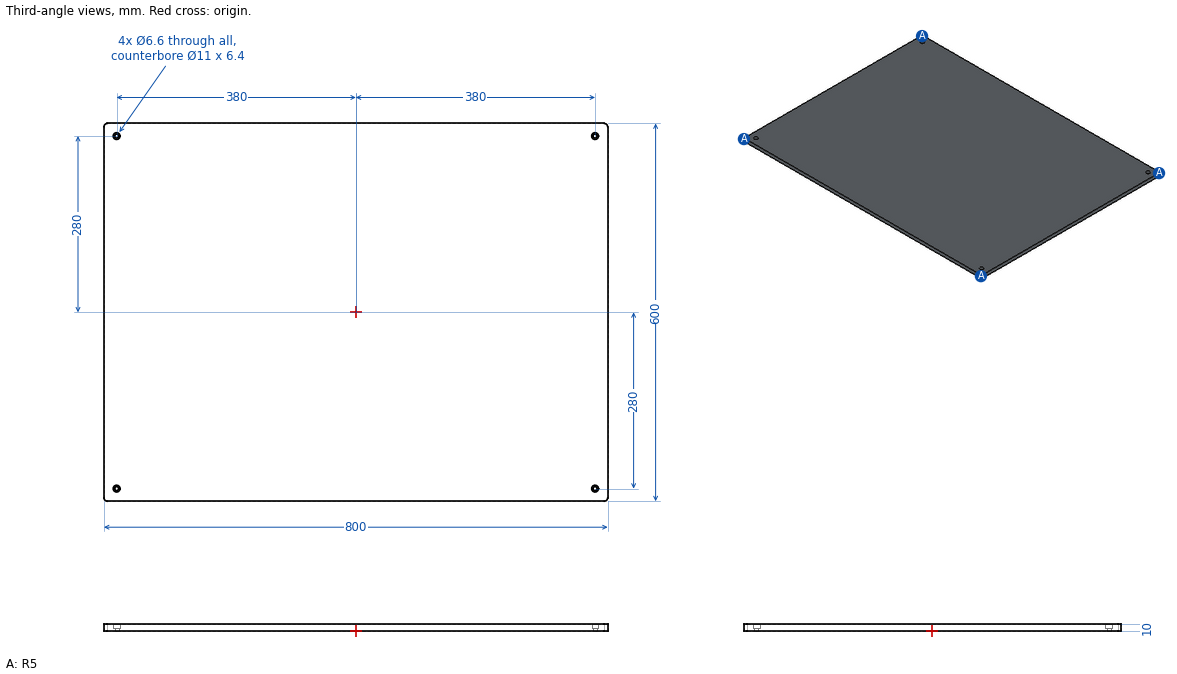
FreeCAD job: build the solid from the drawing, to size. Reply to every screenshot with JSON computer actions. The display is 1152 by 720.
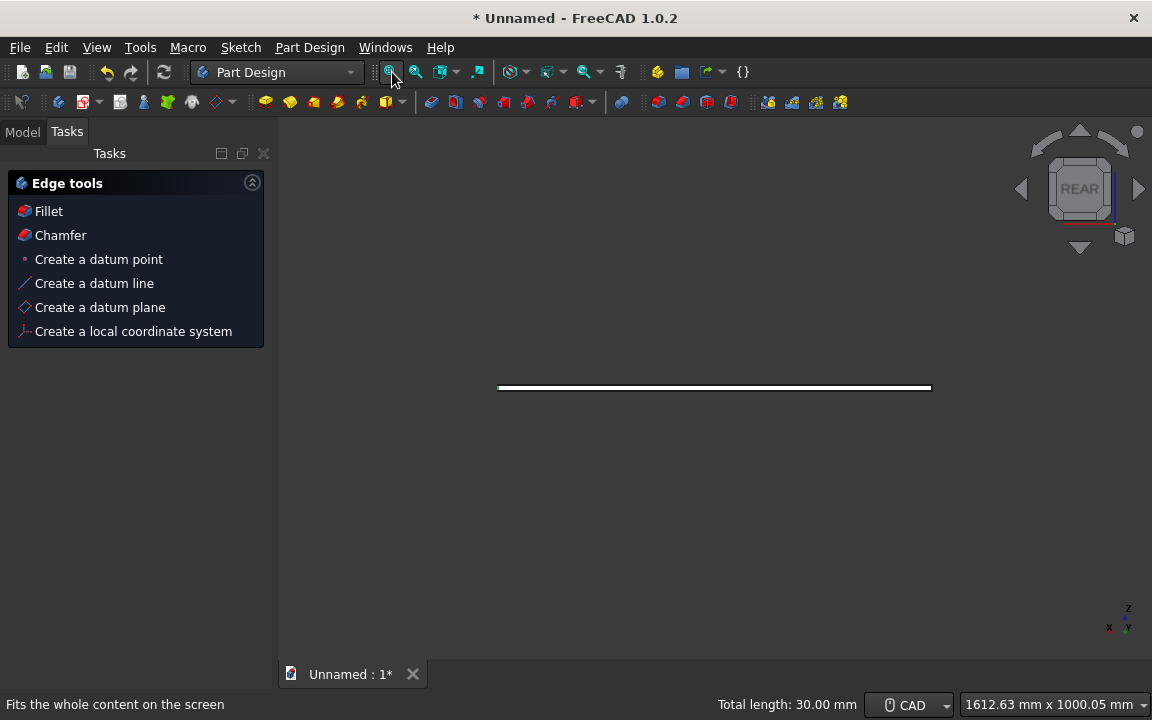
{"action": "scroll", "coordinate": [932, 387], "scroll_direction": "up", "scroll_amount": 10}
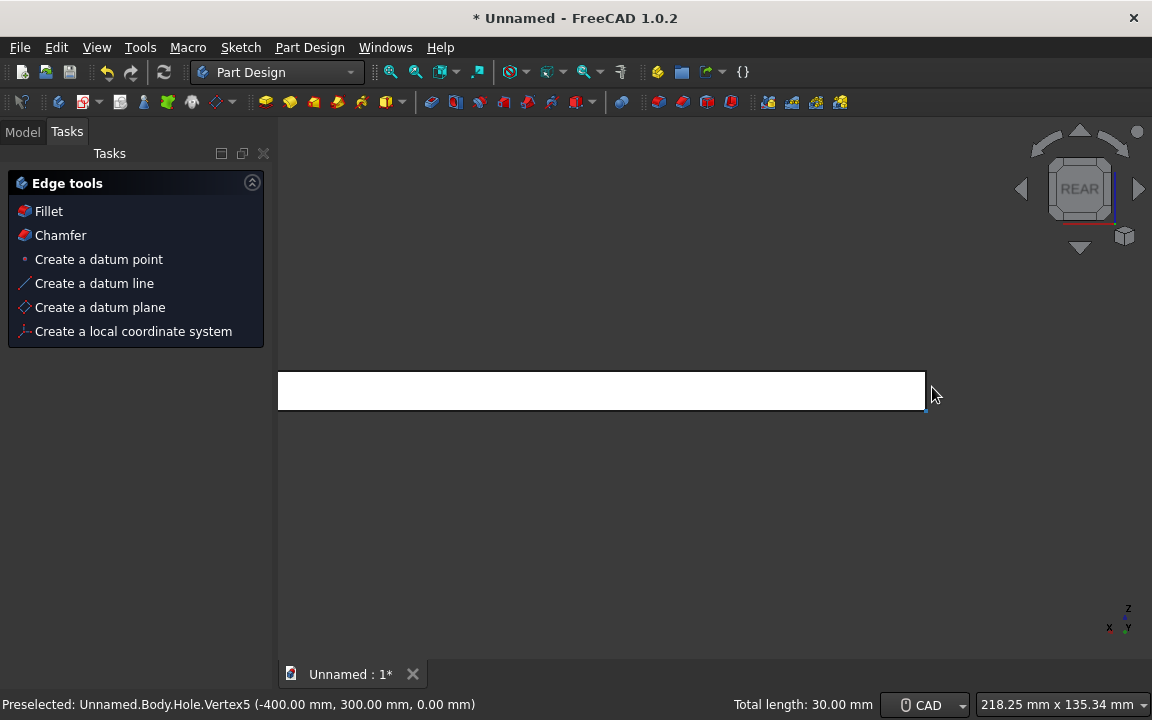
{"action": "left_click", "coordinate": [926, 390], "text": "ctrl"}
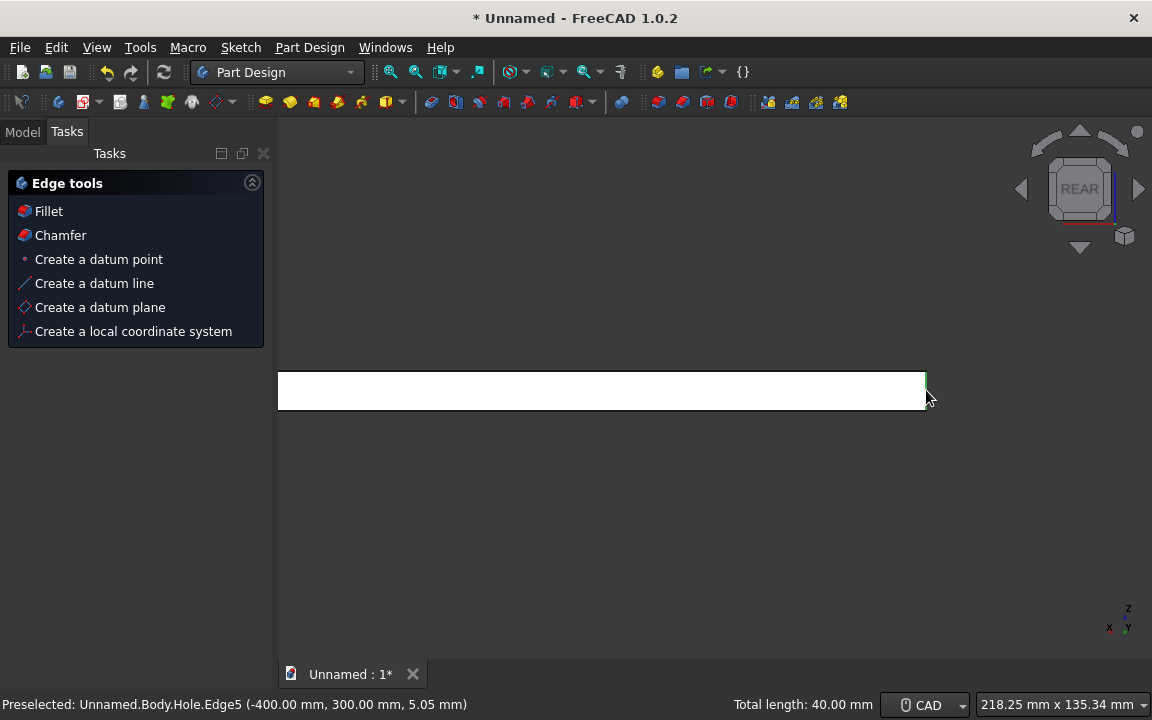
{"action": "left_click", "coordinate": [660, 102]}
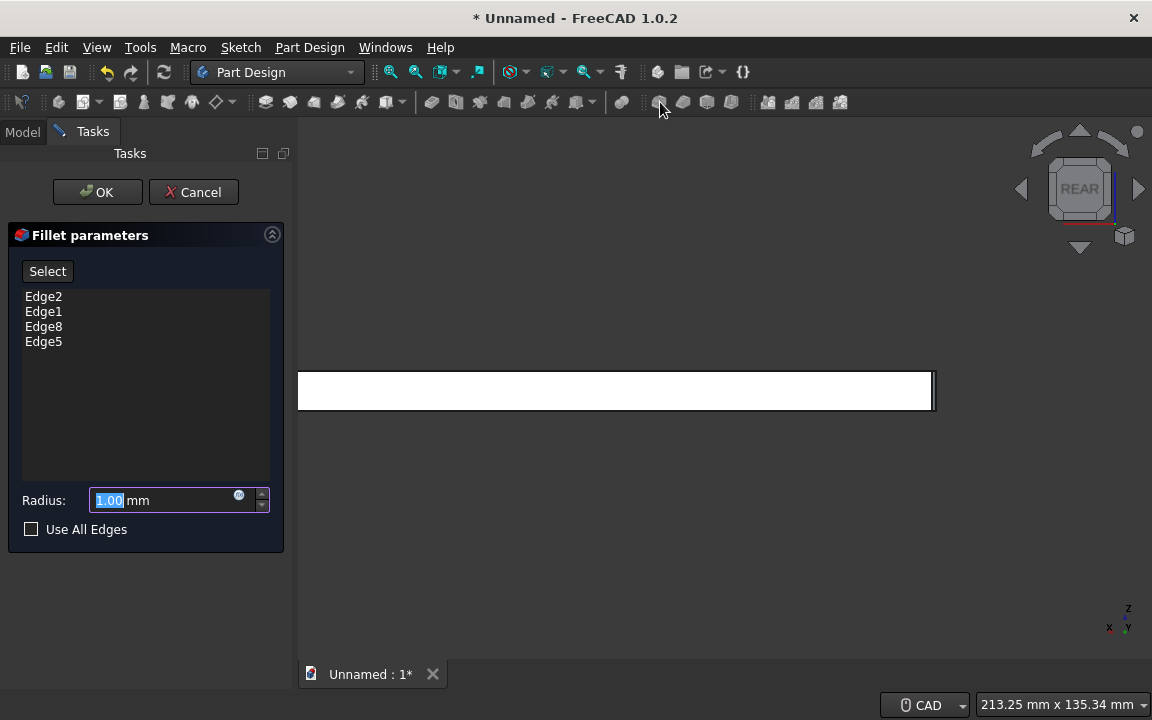
{"action": "type", "text": "5"}
{"action": "key", "text": "Tab"}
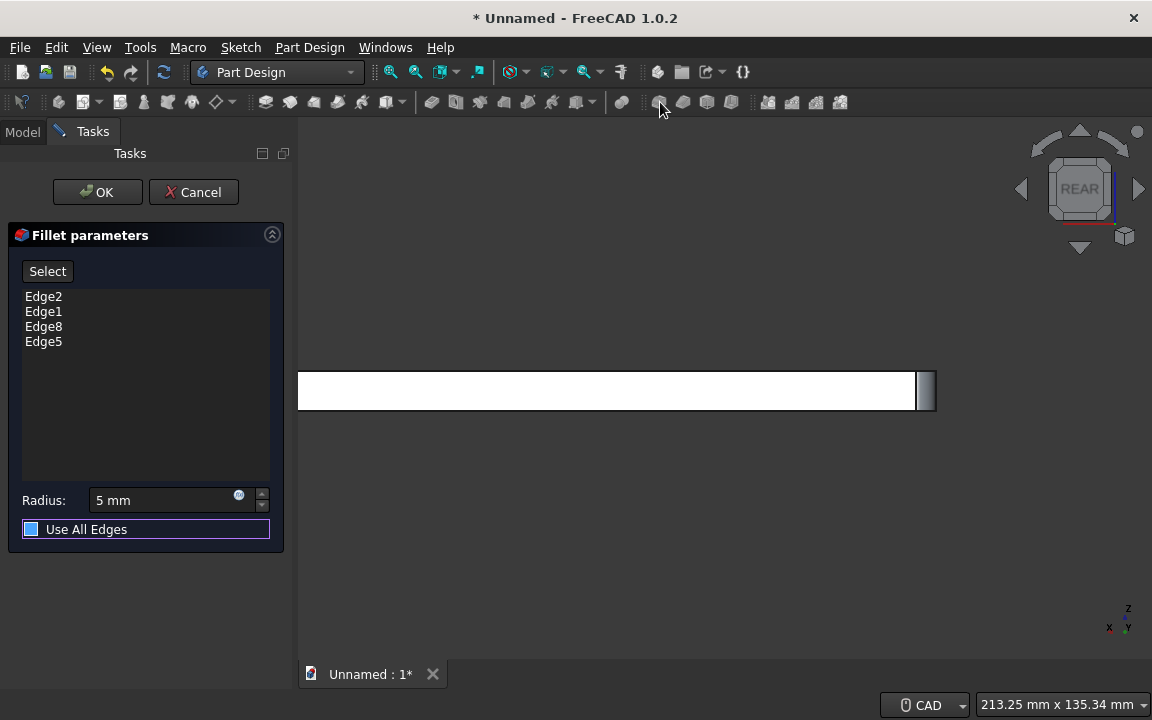
{"action": "left_click", "coordinate": [98, 192]}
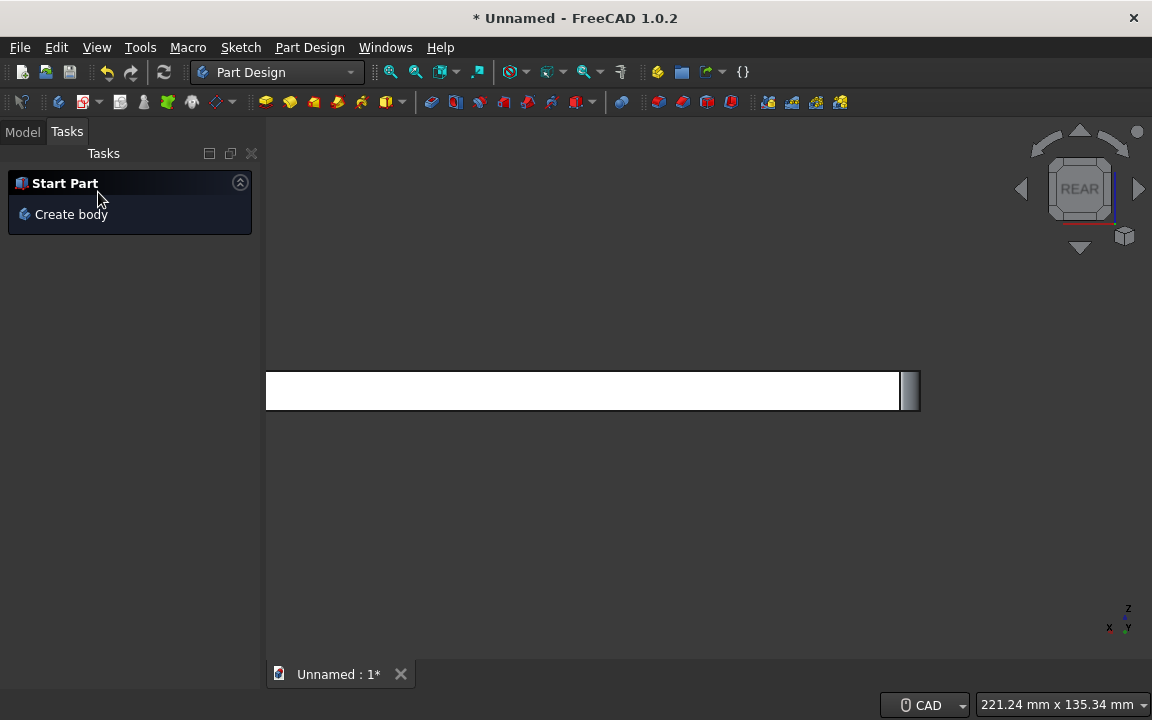
{"action": "key", "text": "0"}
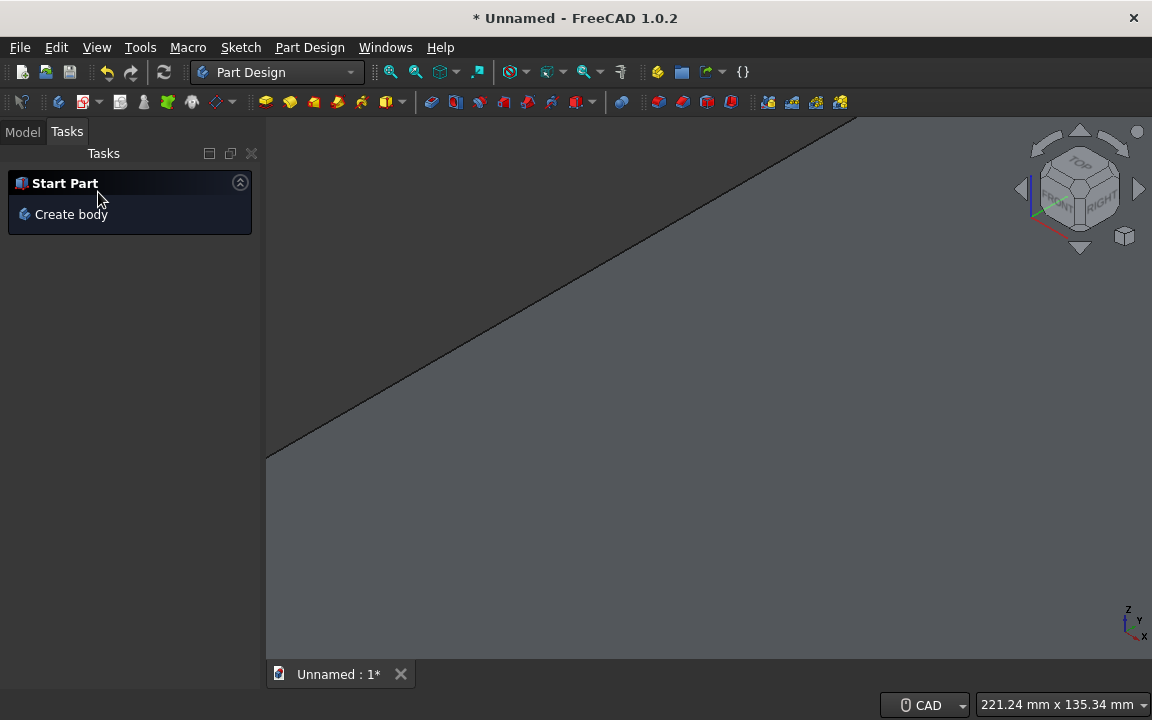
{"action": "key", "text": "v f"}